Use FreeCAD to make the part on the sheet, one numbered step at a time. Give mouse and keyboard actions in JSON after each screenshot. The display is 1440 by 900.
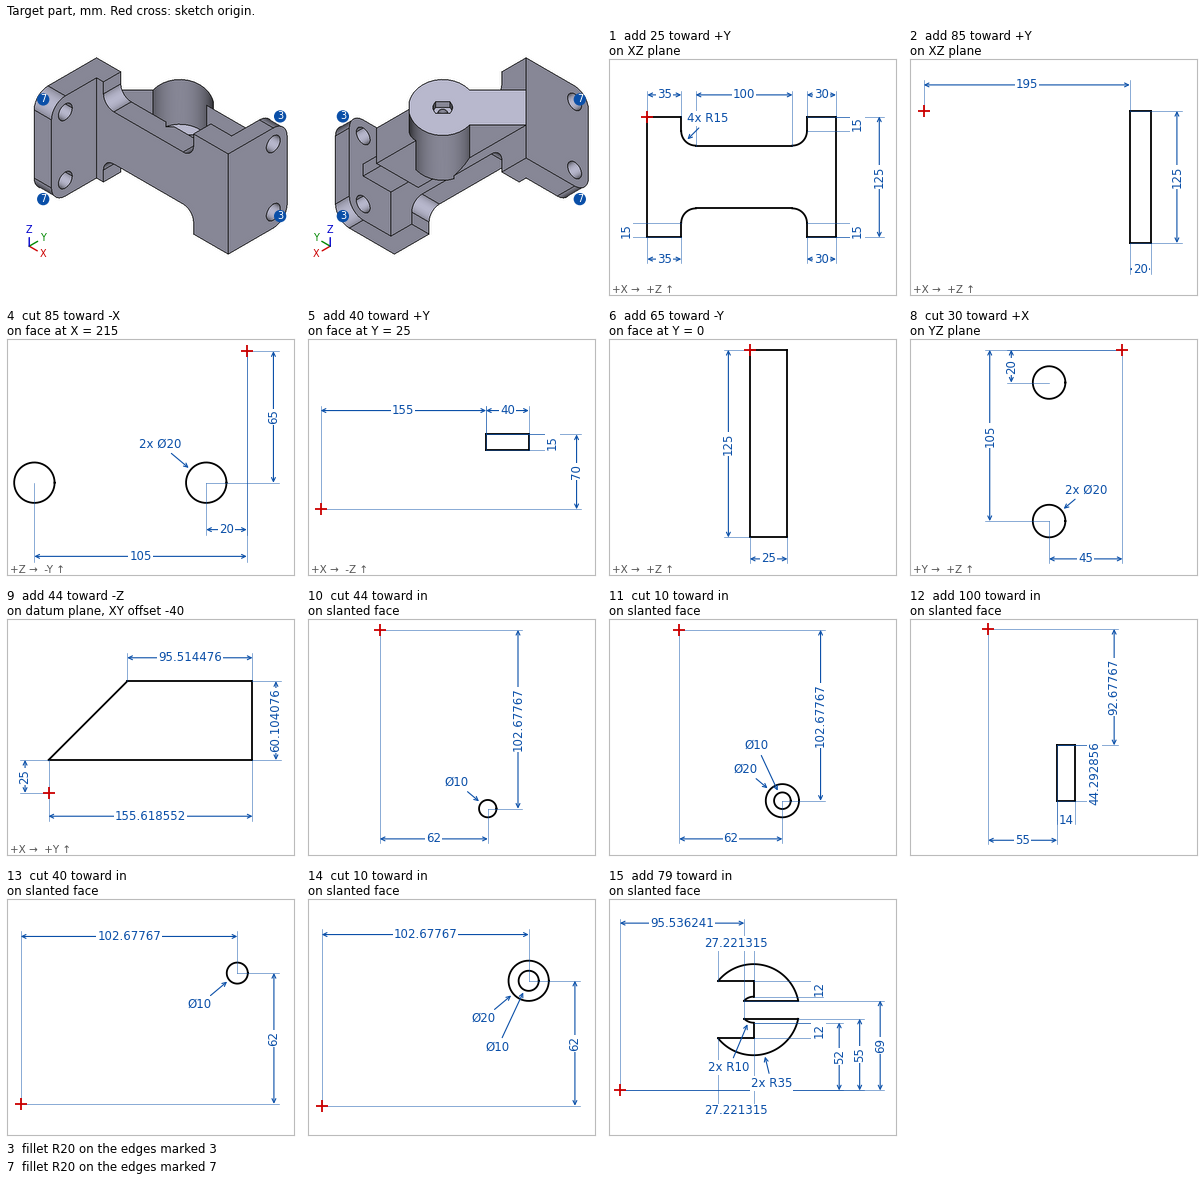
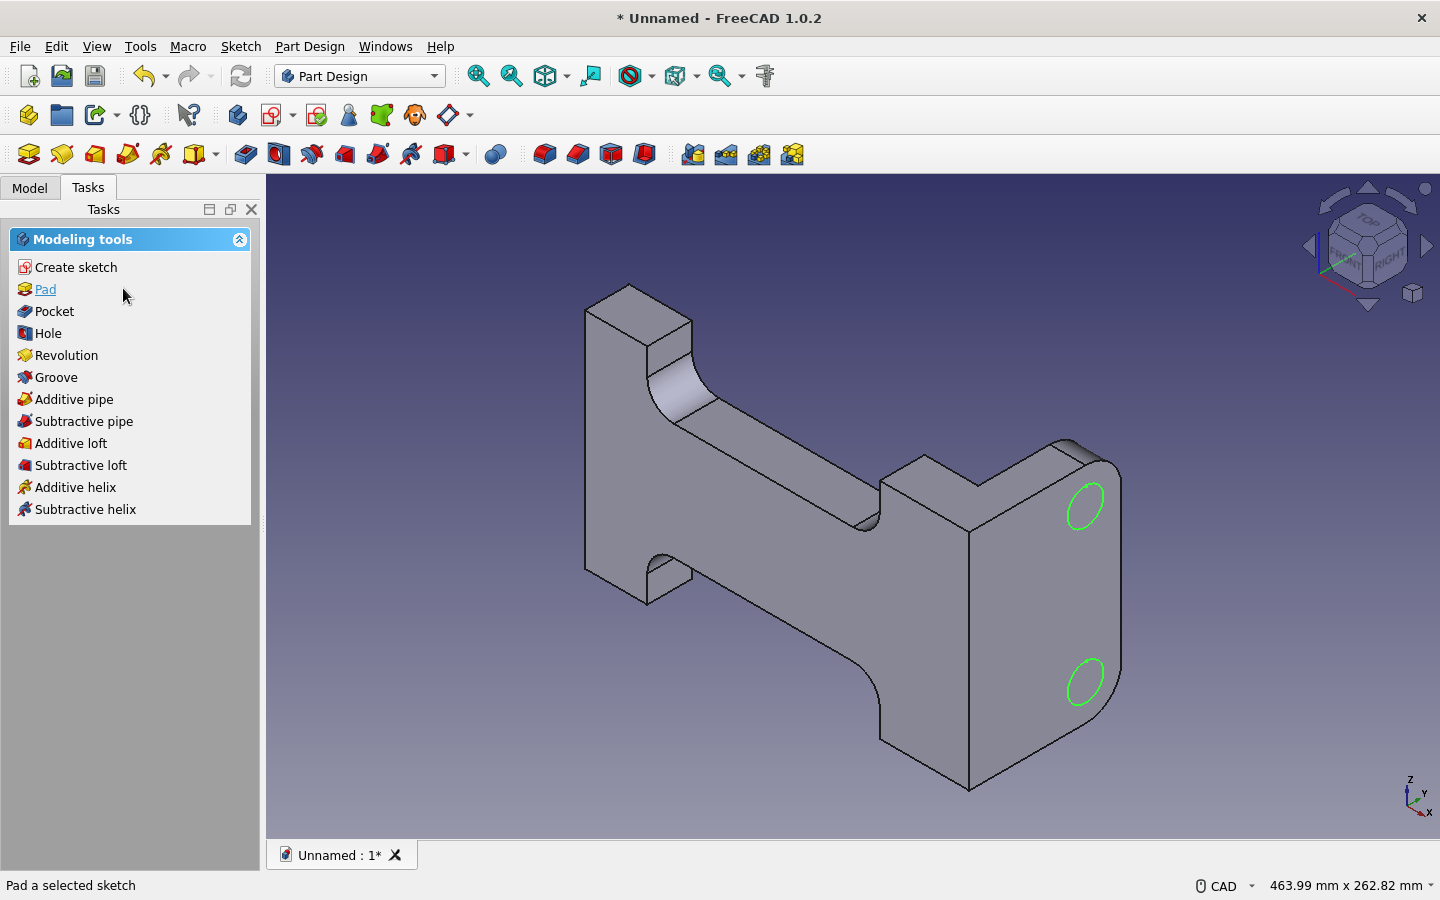
{"action": "left_click", "coordinate": [246, 154]}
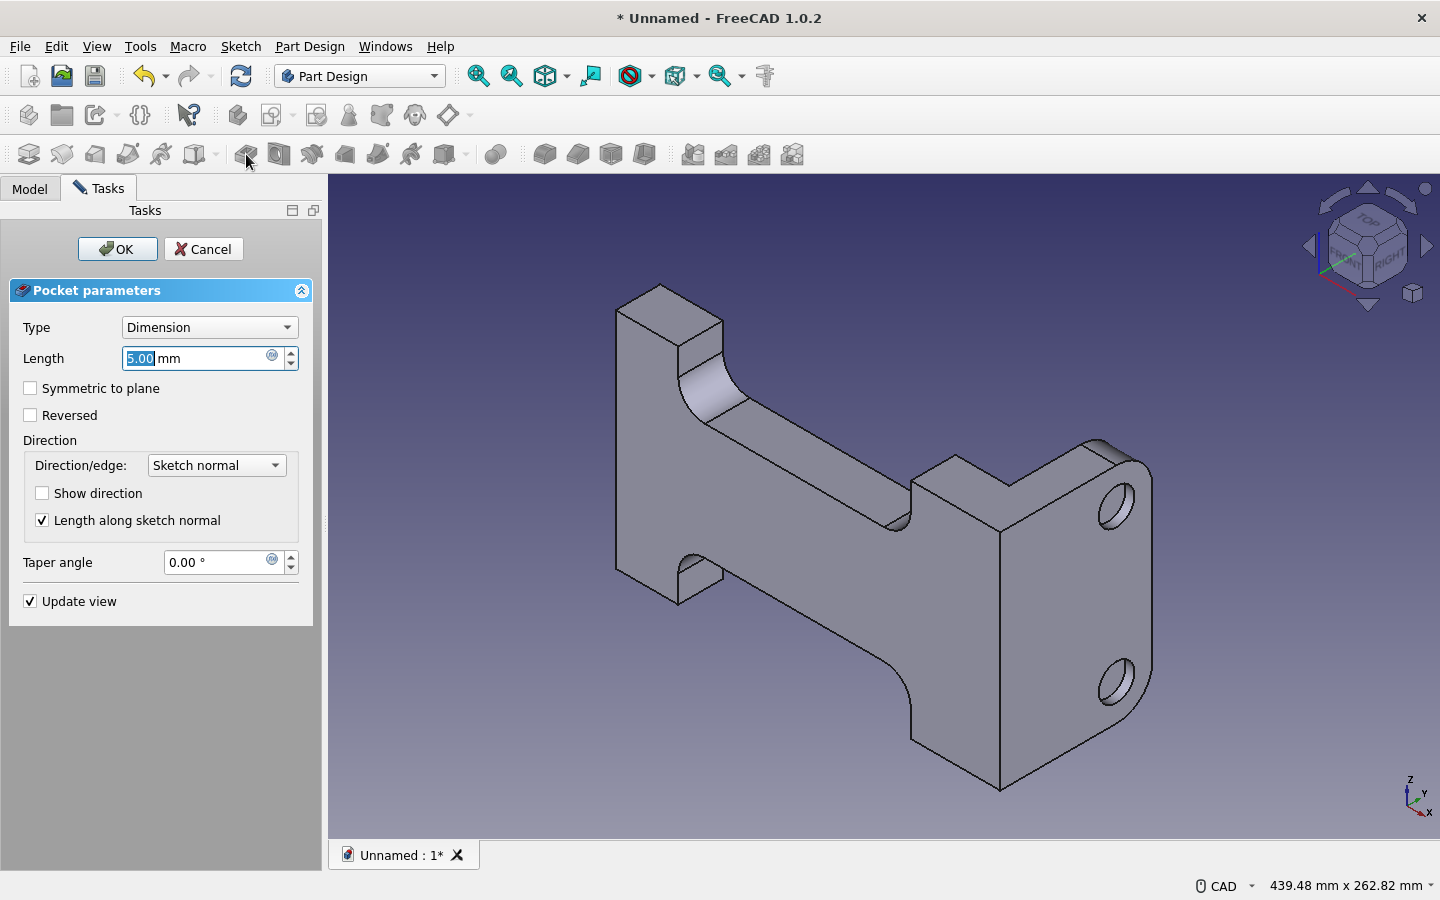
{"action": "type", "text": "85"}
{"action": "key", "text": "Tab"}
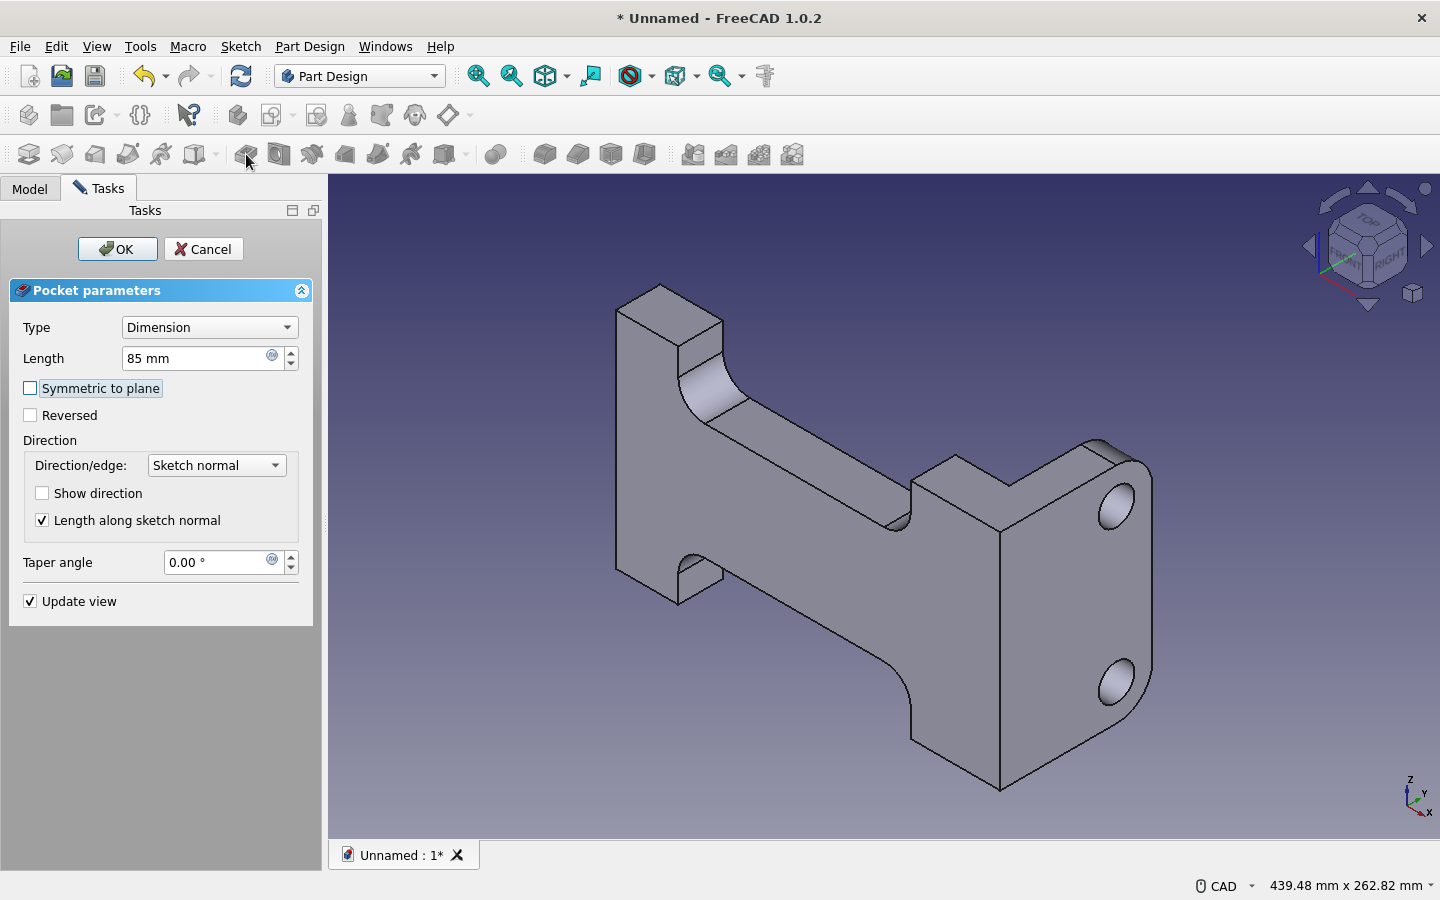
{"action": "left_click", "coordinate": [118, 249]}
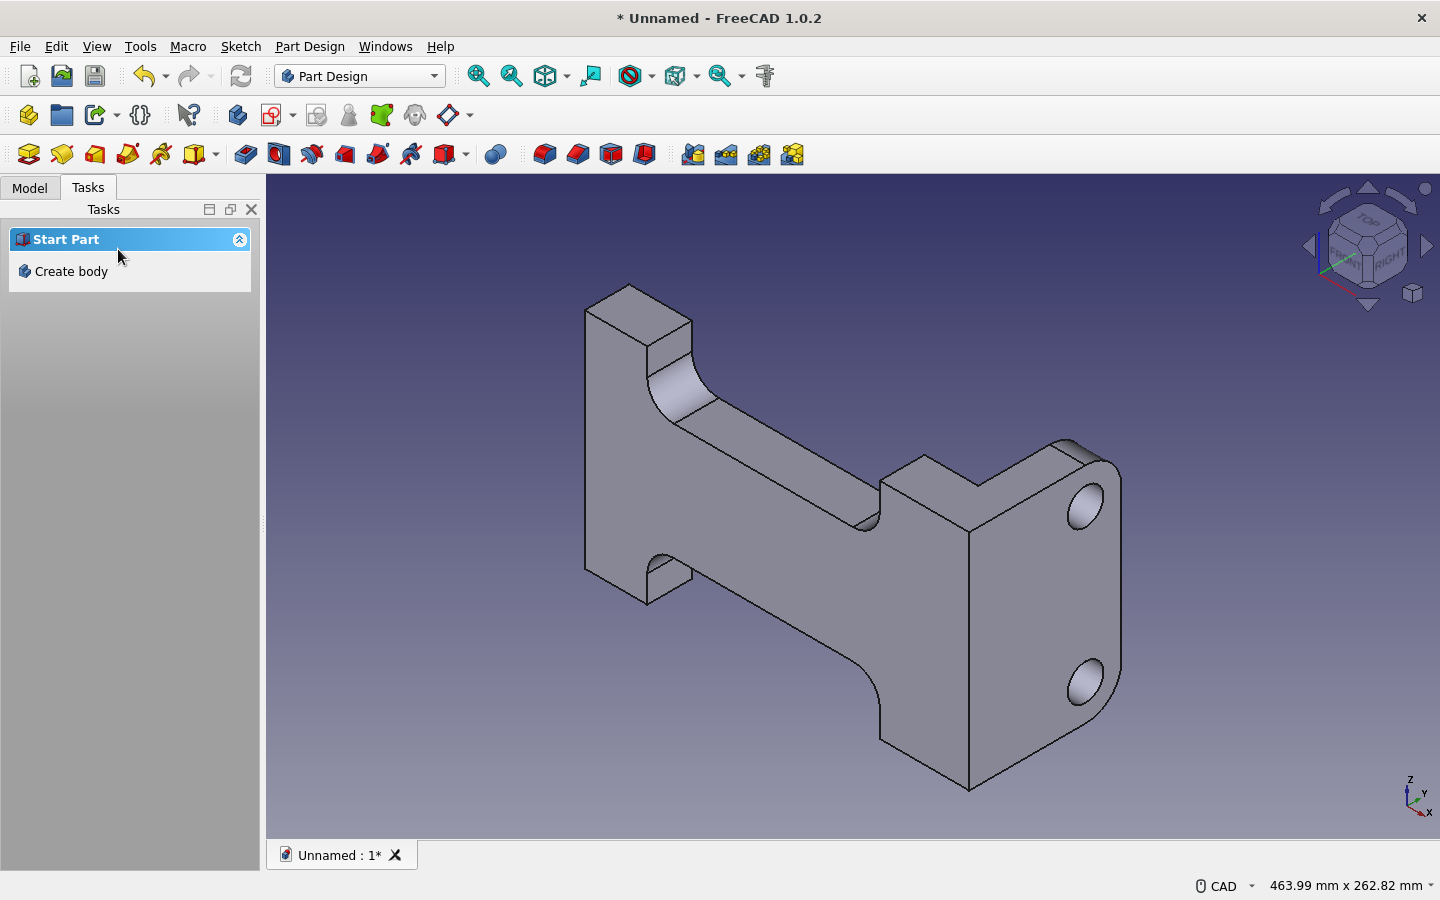
{"action": "key", "text": "4"}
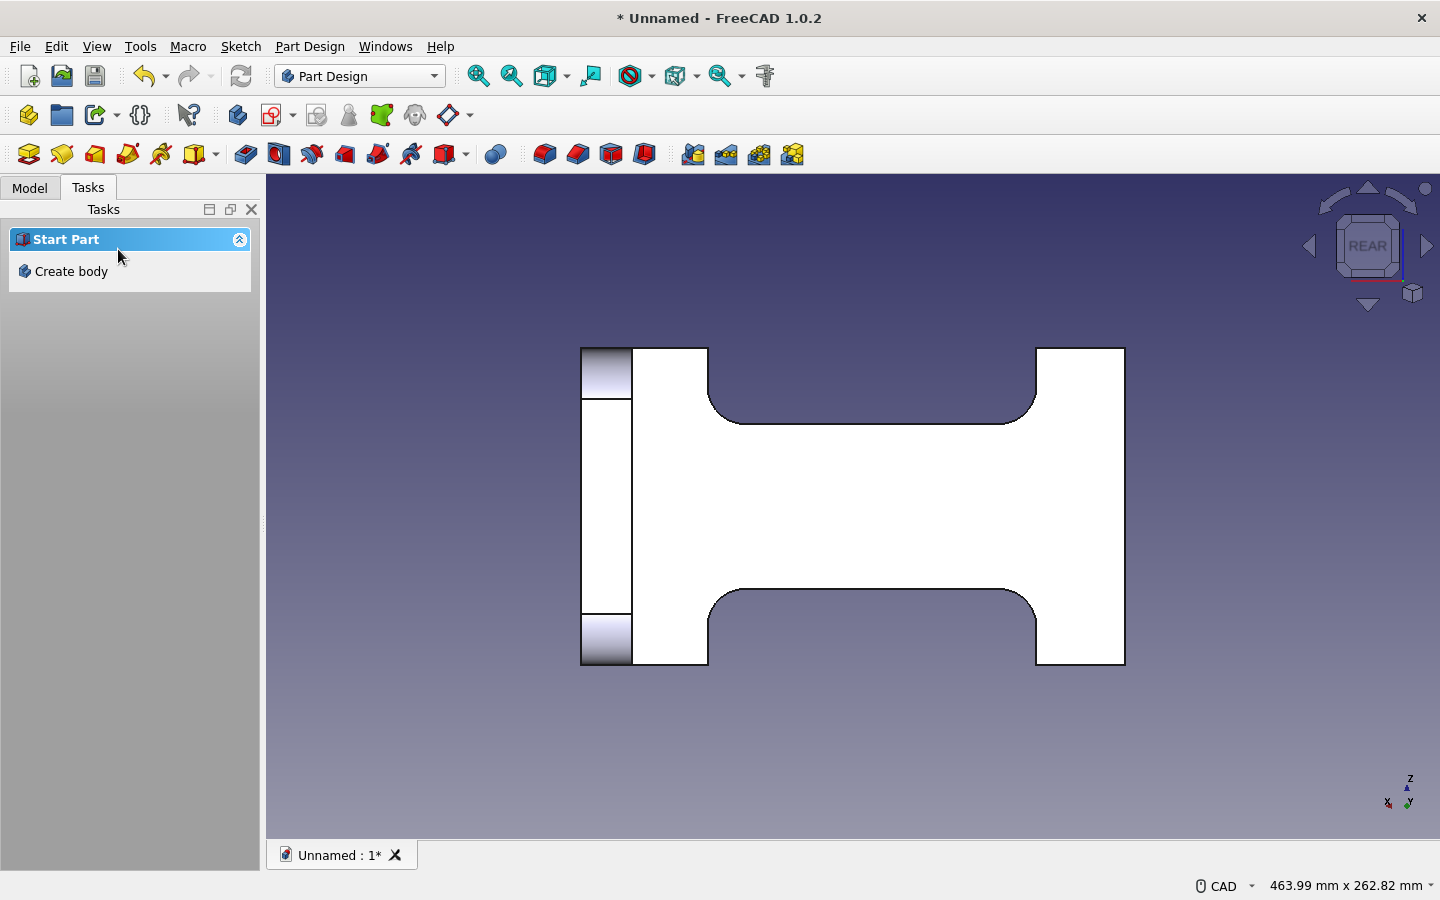
{"action": "left_click", "coordinate": [1019, 505]}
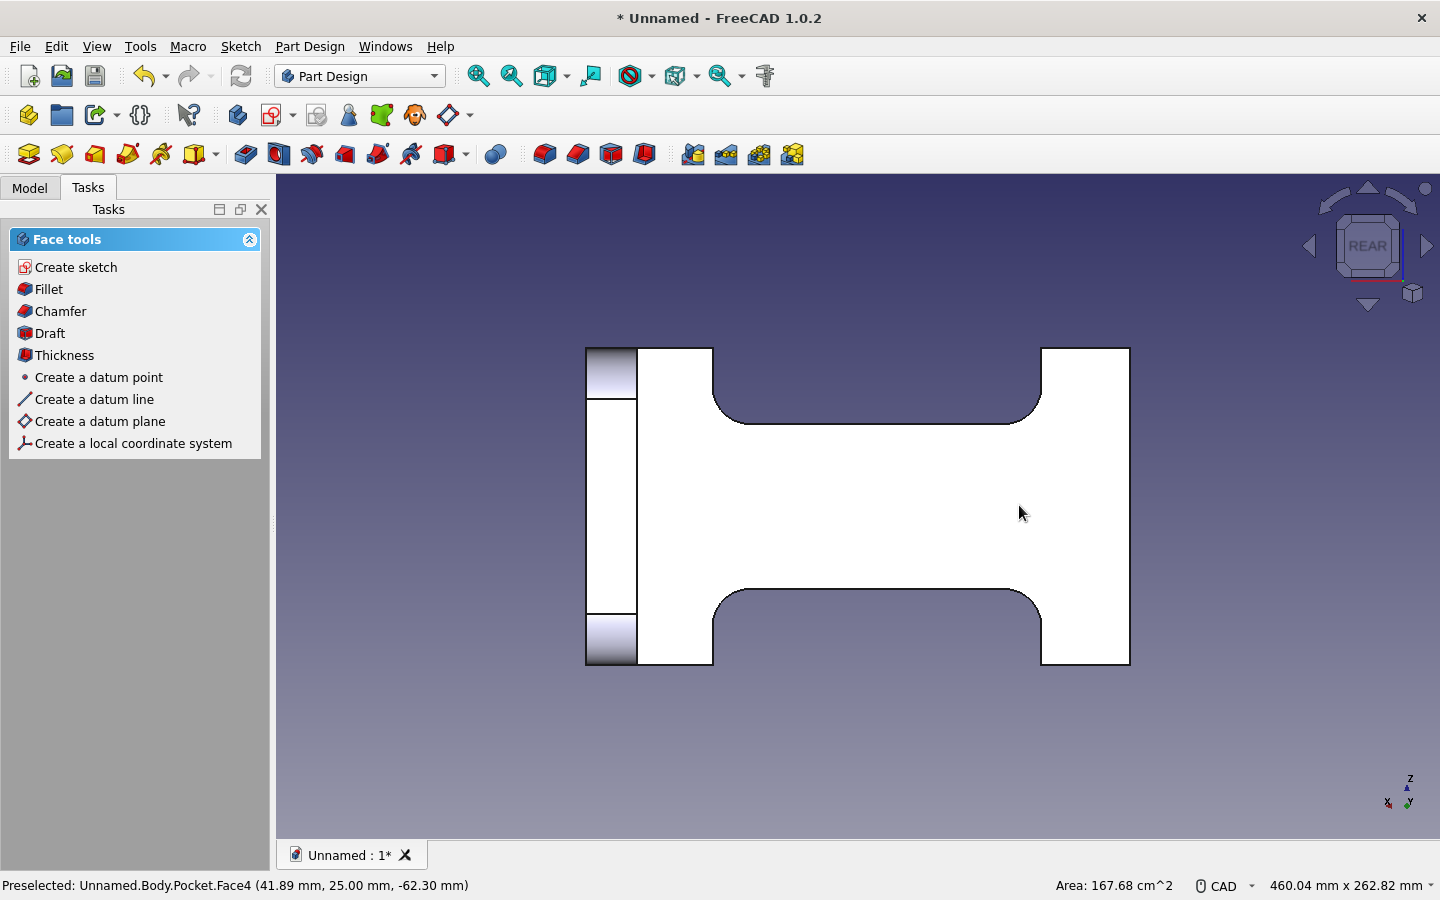
{"action": "left_click", "coordinate": [270, 116]}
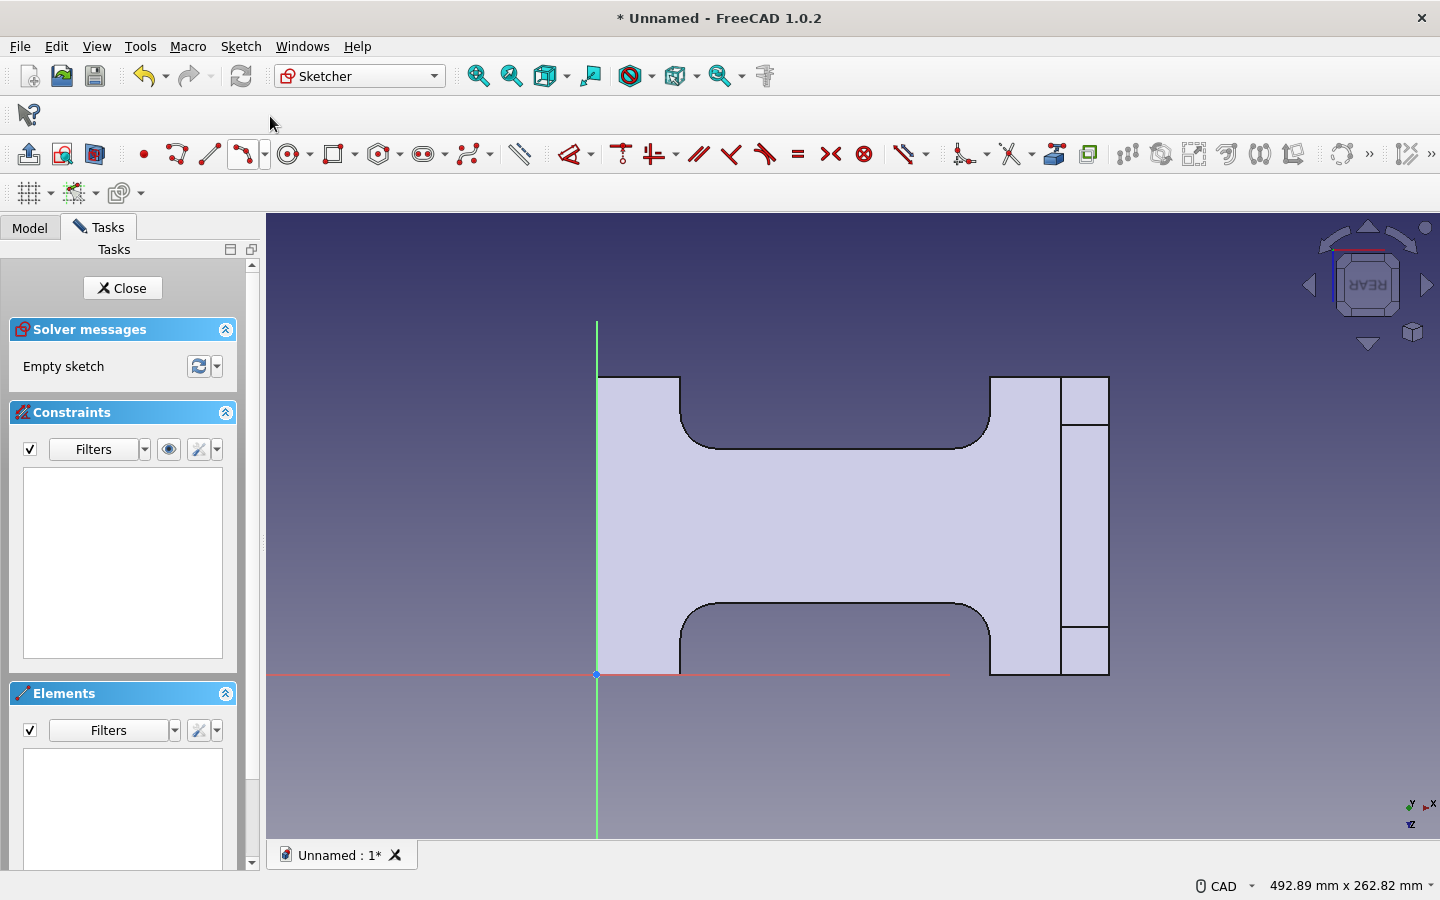
{"action": "left_click", "coordinate": [95, 154]}